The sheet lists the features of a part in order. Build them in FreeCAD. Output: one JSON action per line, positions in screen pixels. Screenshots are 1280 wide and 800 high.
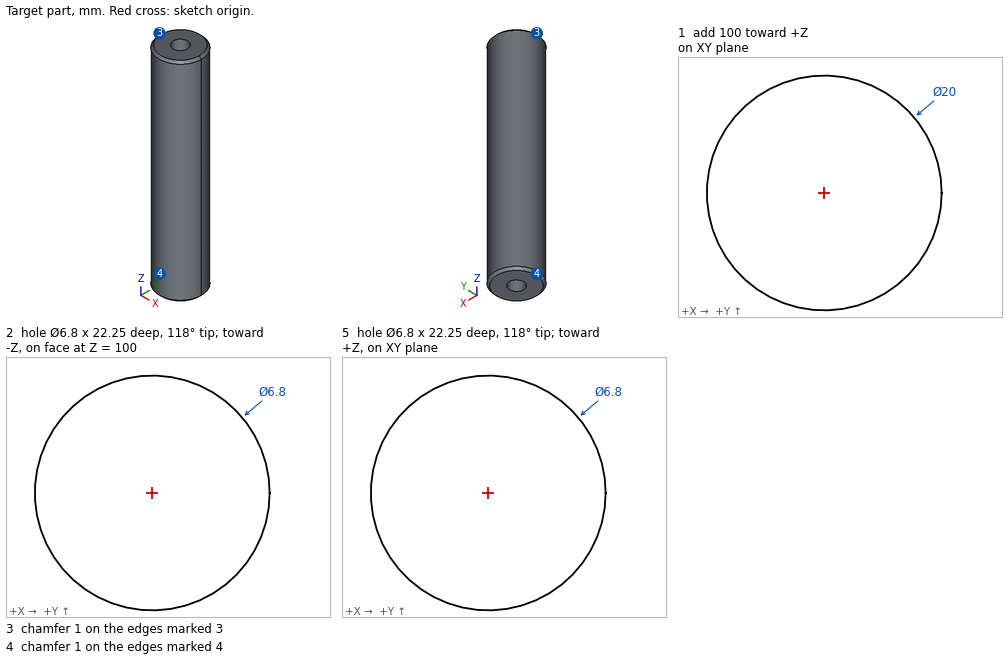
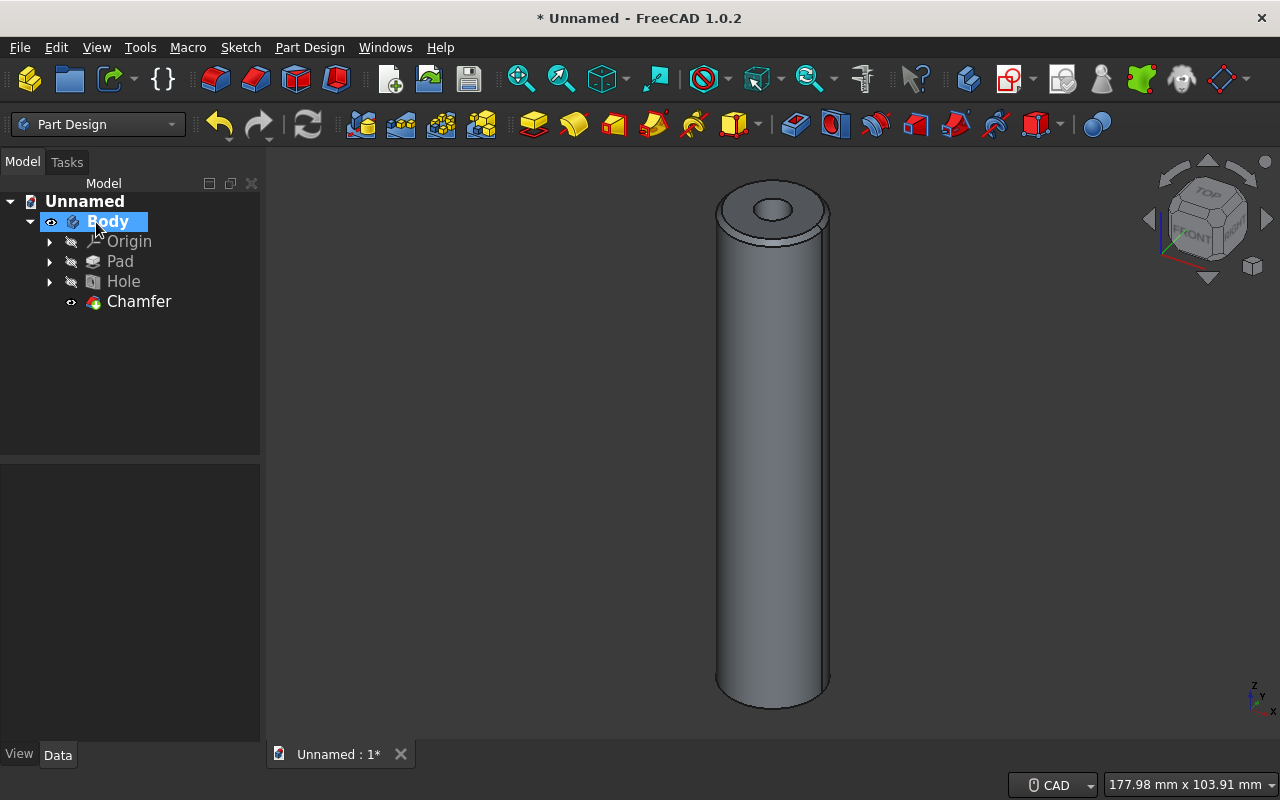
{"action": "key", "text": "0"}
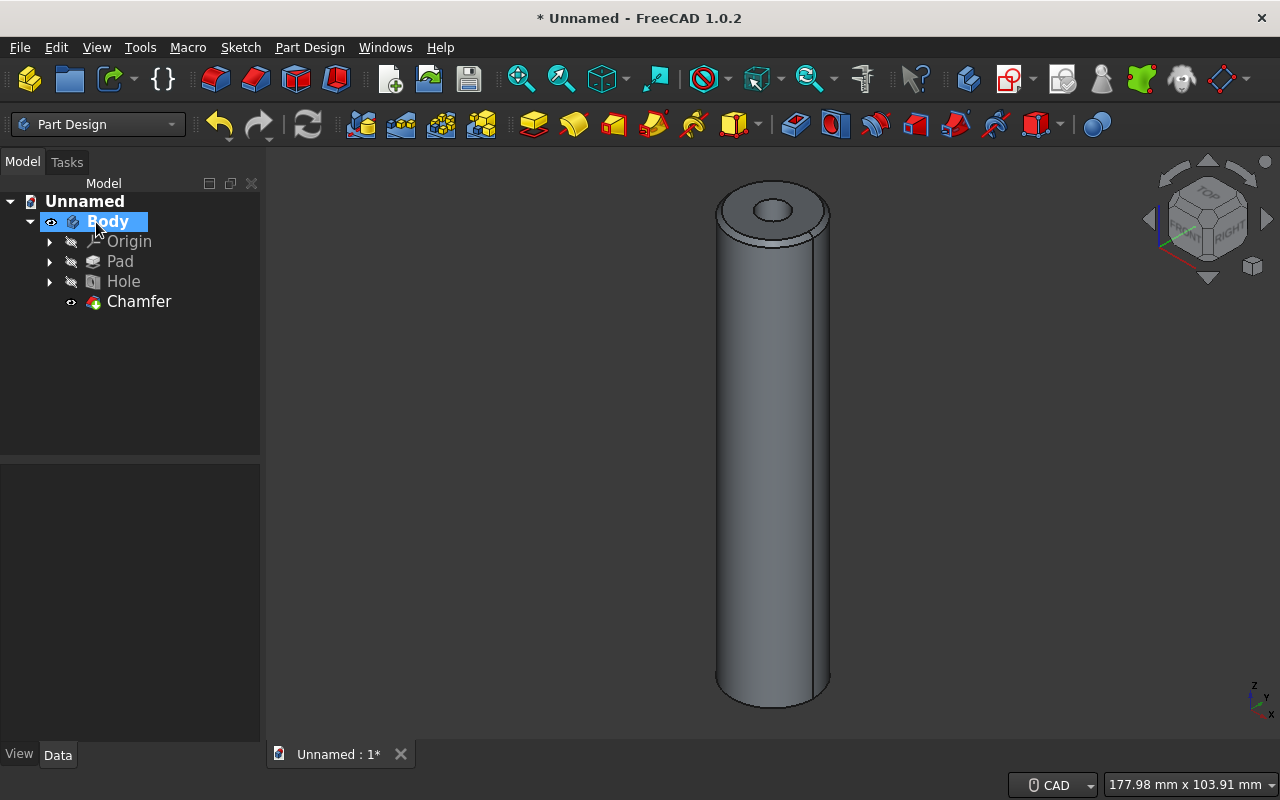
{"action": "key", "text": "2"}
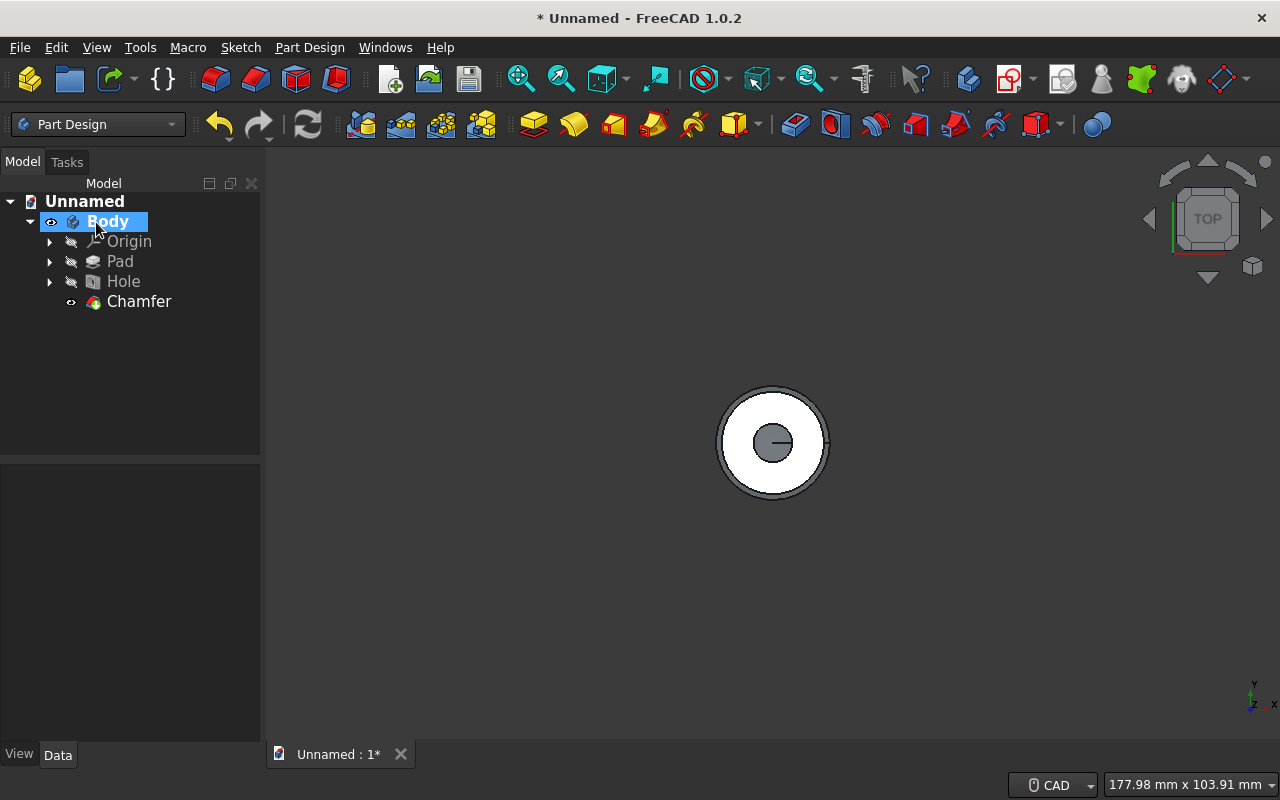
{"action": "key", "text": "v f"}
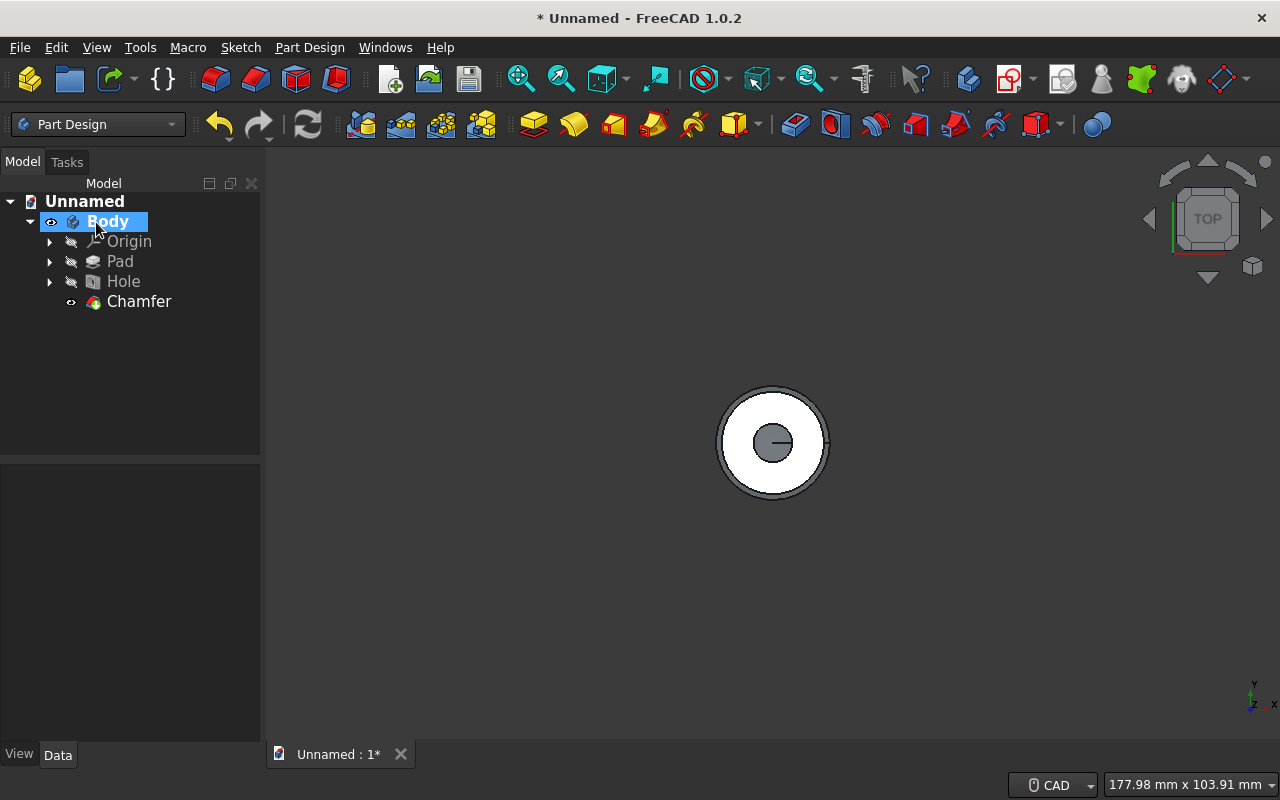
{"action": "key", "text": "1"}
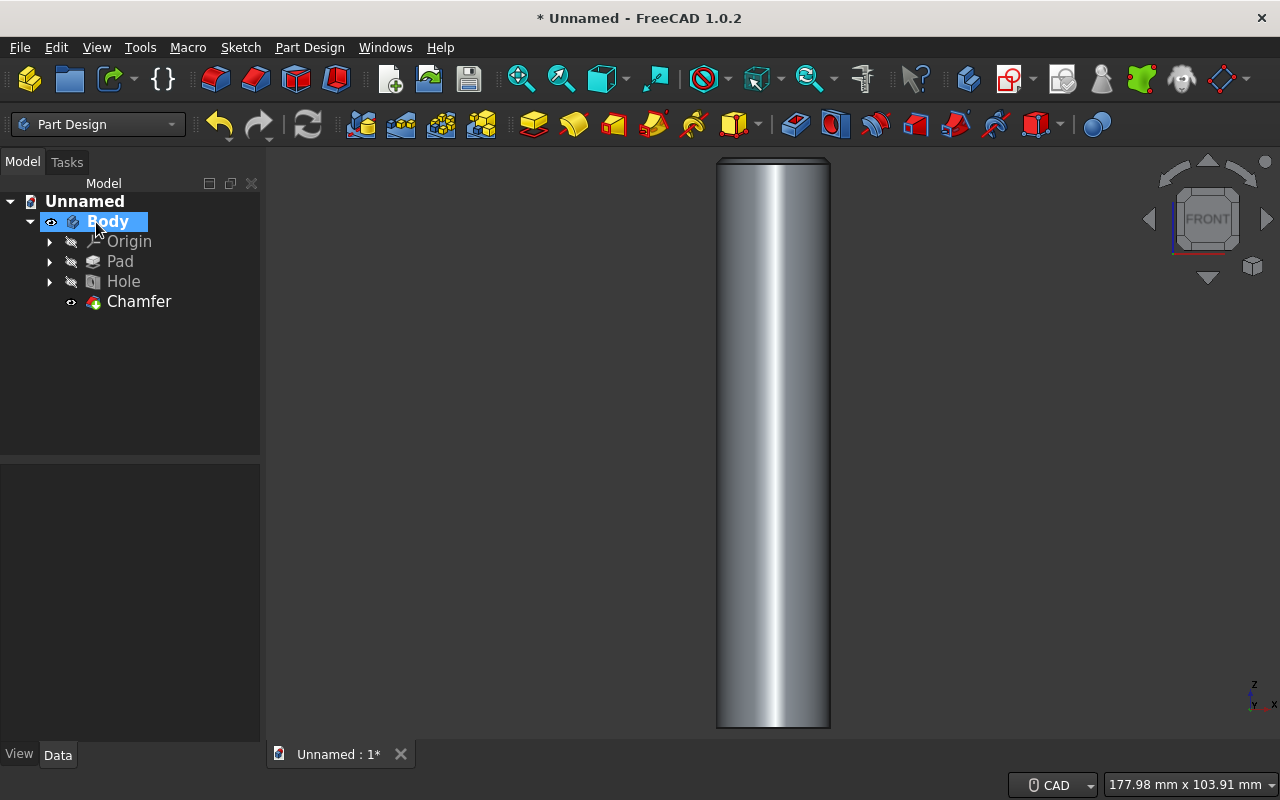
{"action": "key", "text": "3"}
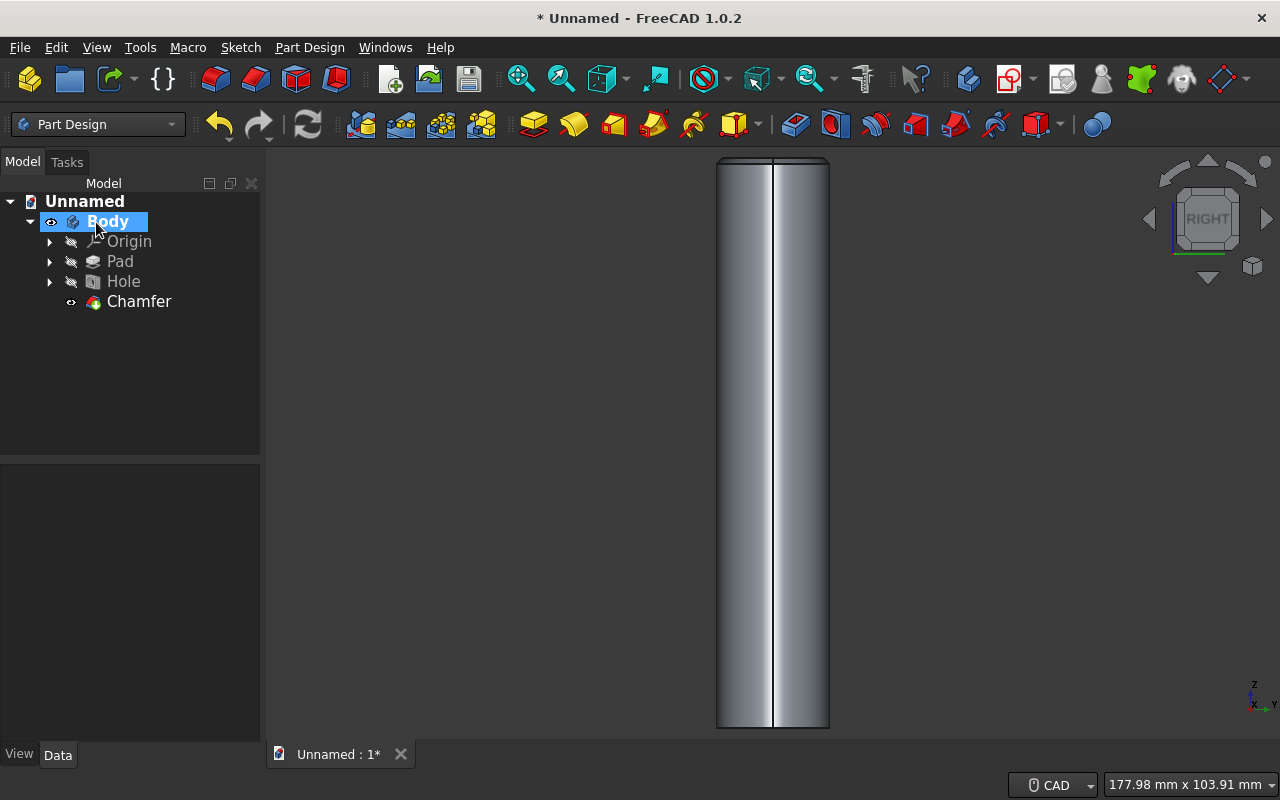
{"action": "key", "text": "5"}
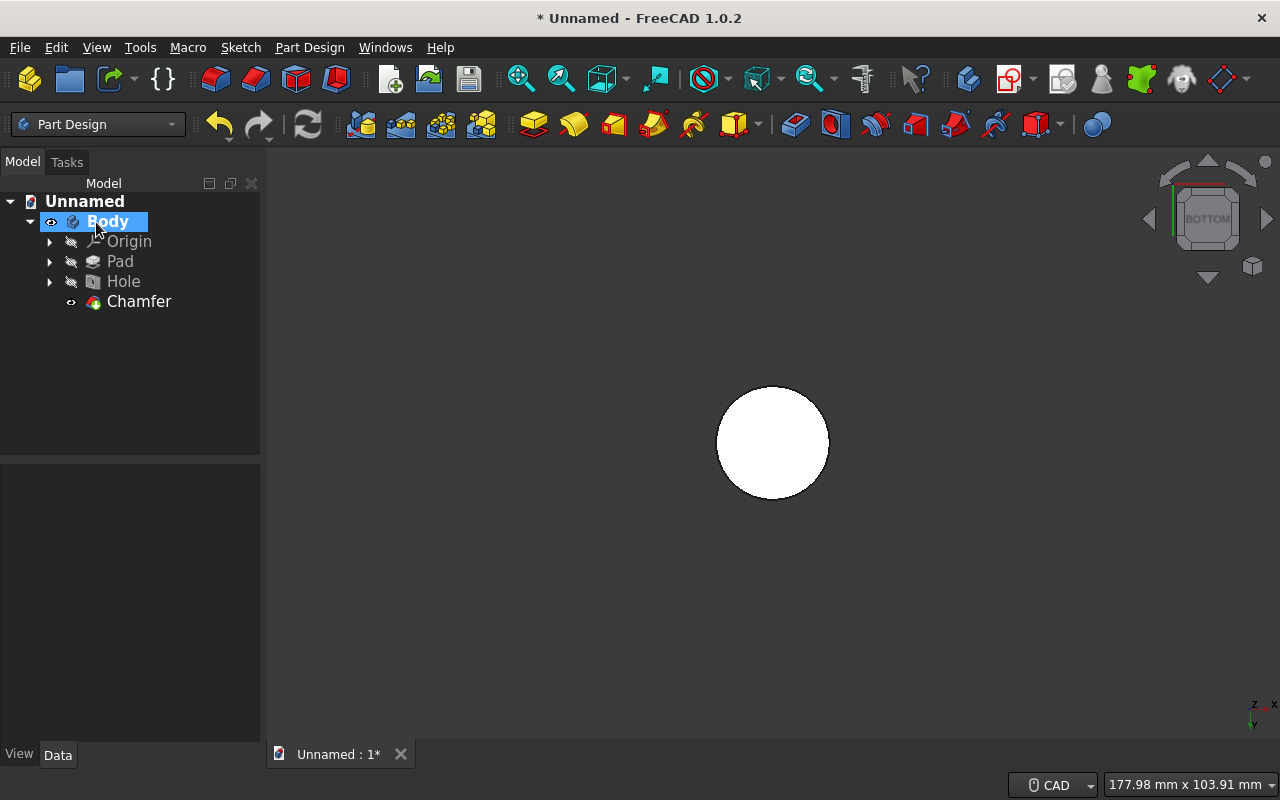
{"action": "left_click", "coordinate": [522, 80]}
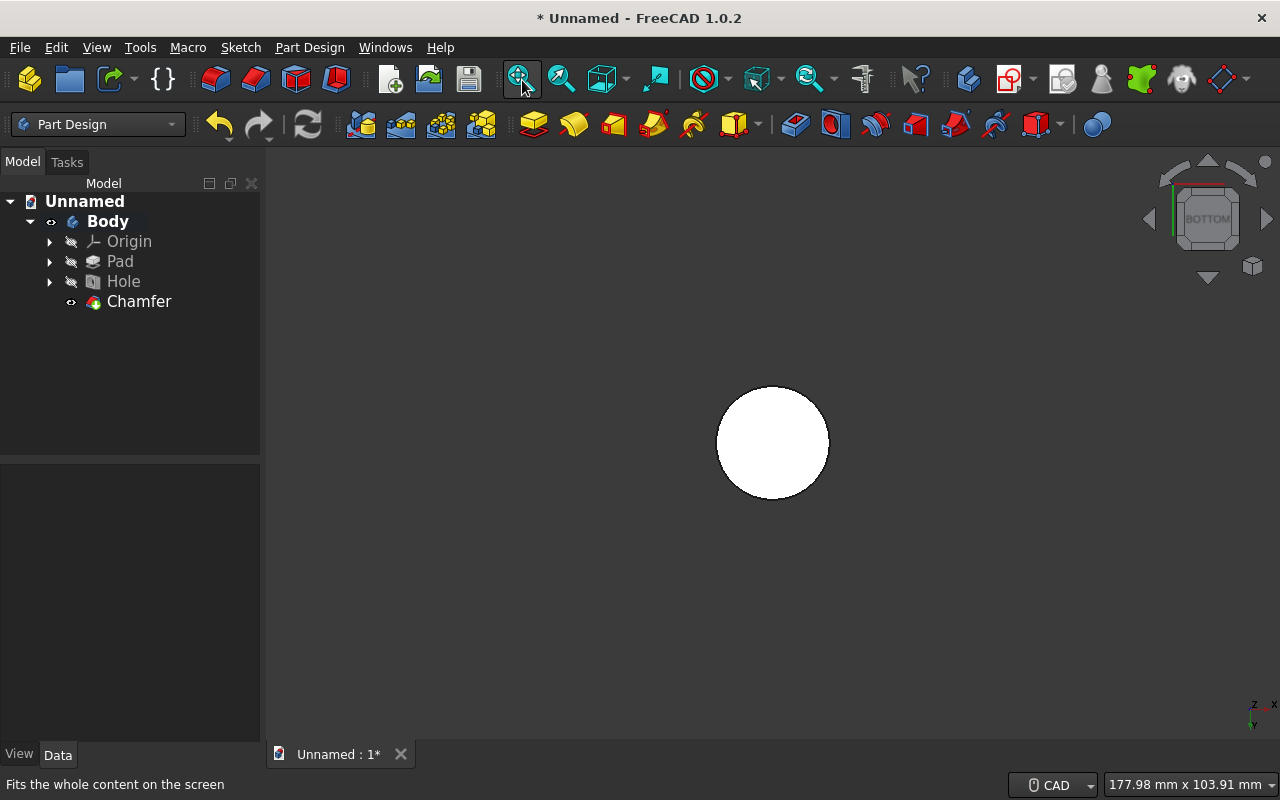
{"action": "left_click", "coordinate": [716, 442]}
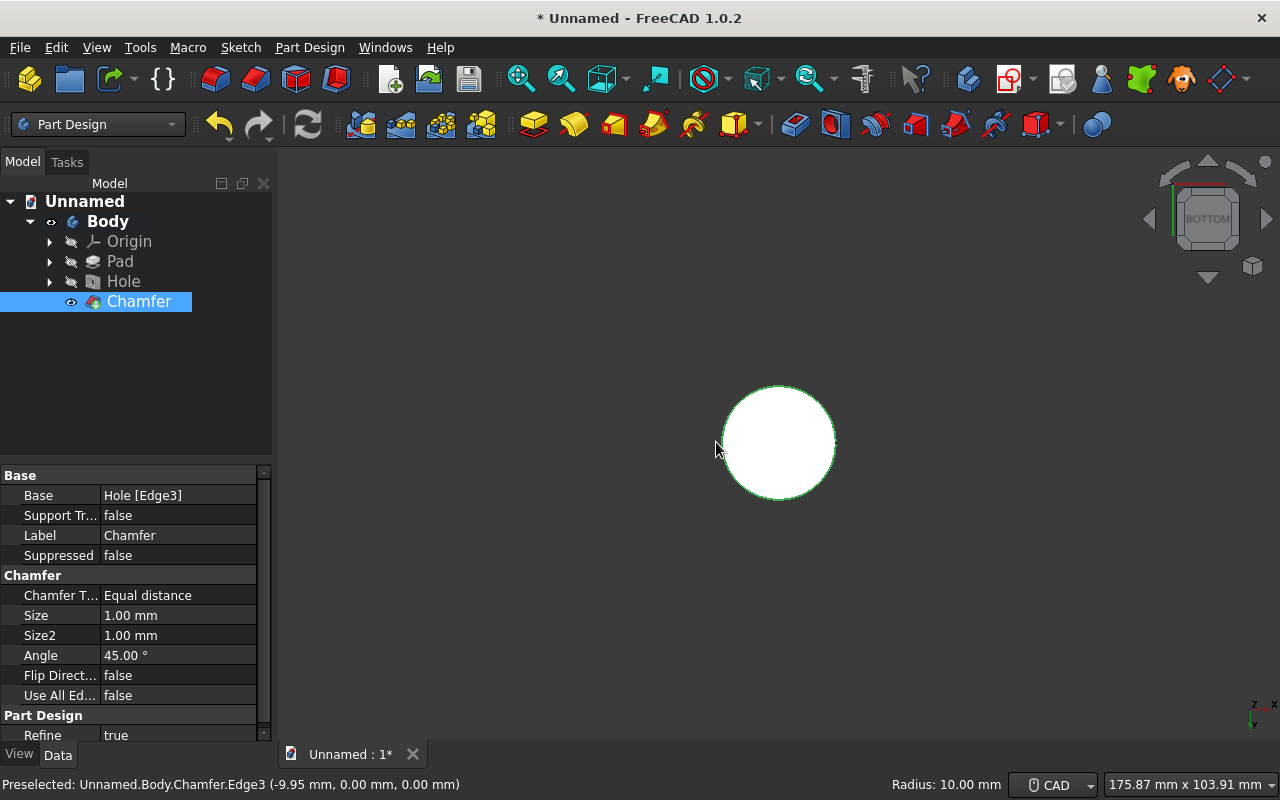
{"action": "left_click", "coordinate": [256, 80]}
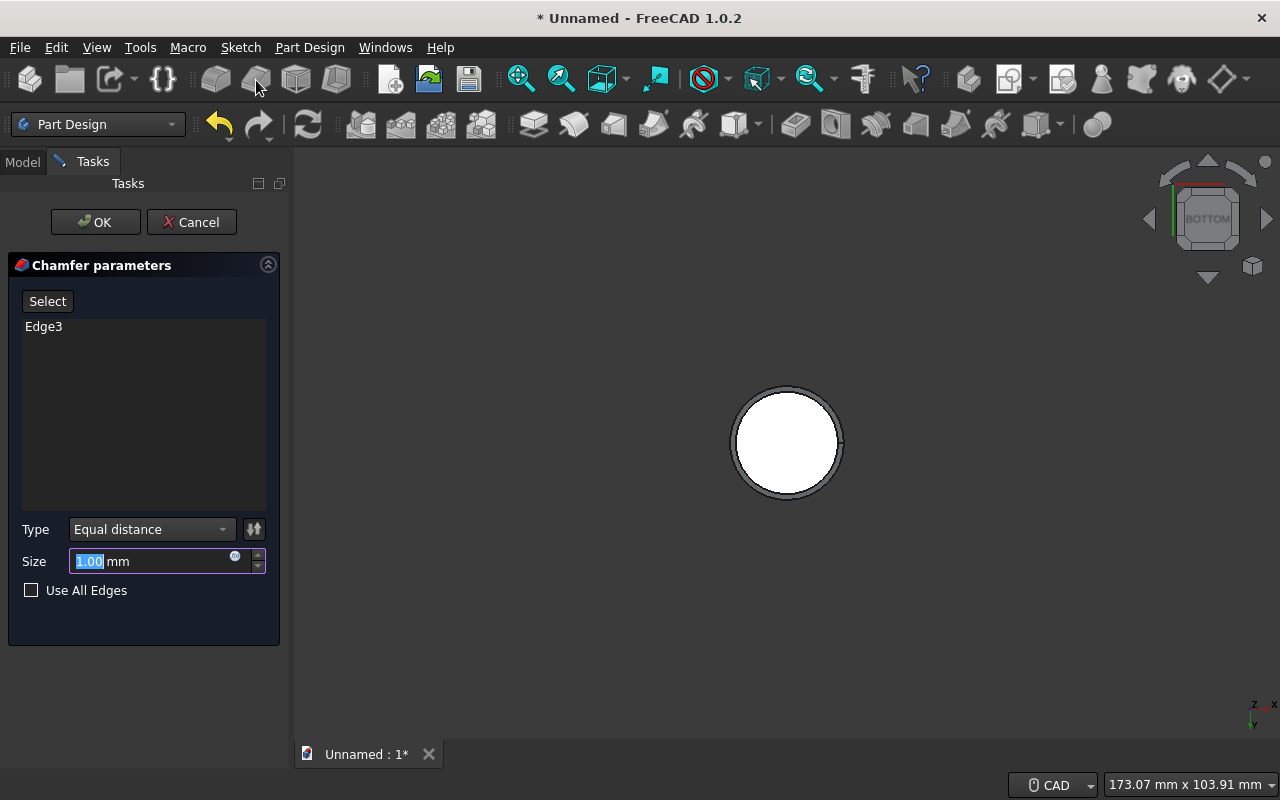
{"action": "type", "text": "1"}
{"action": "key", "text": "Tab"}